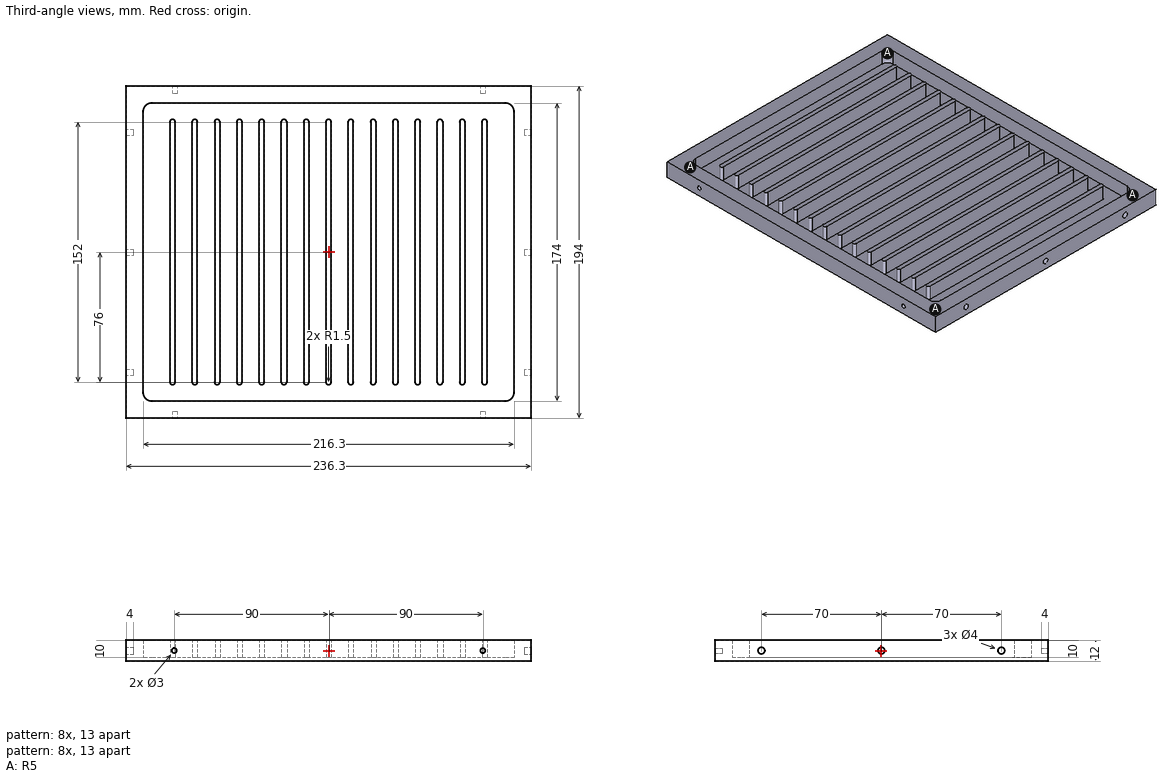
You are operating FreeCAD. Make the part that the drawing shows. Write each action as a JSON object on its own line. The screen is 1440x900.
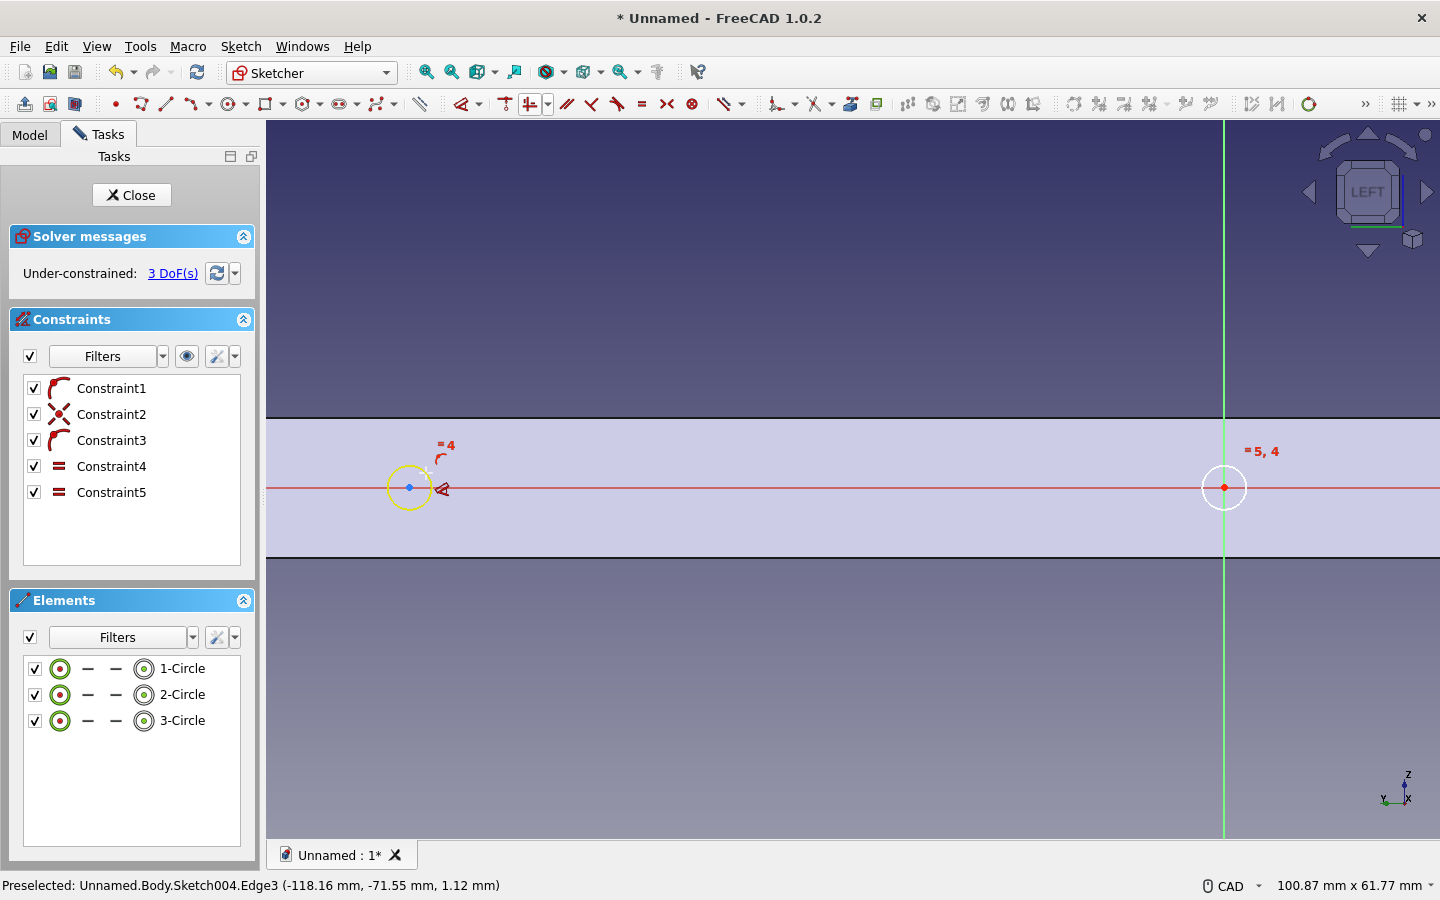
{"action": "left_click", "coordinate": [425, 472]}
{"action": "left_click", "coordinate": [447, 449]}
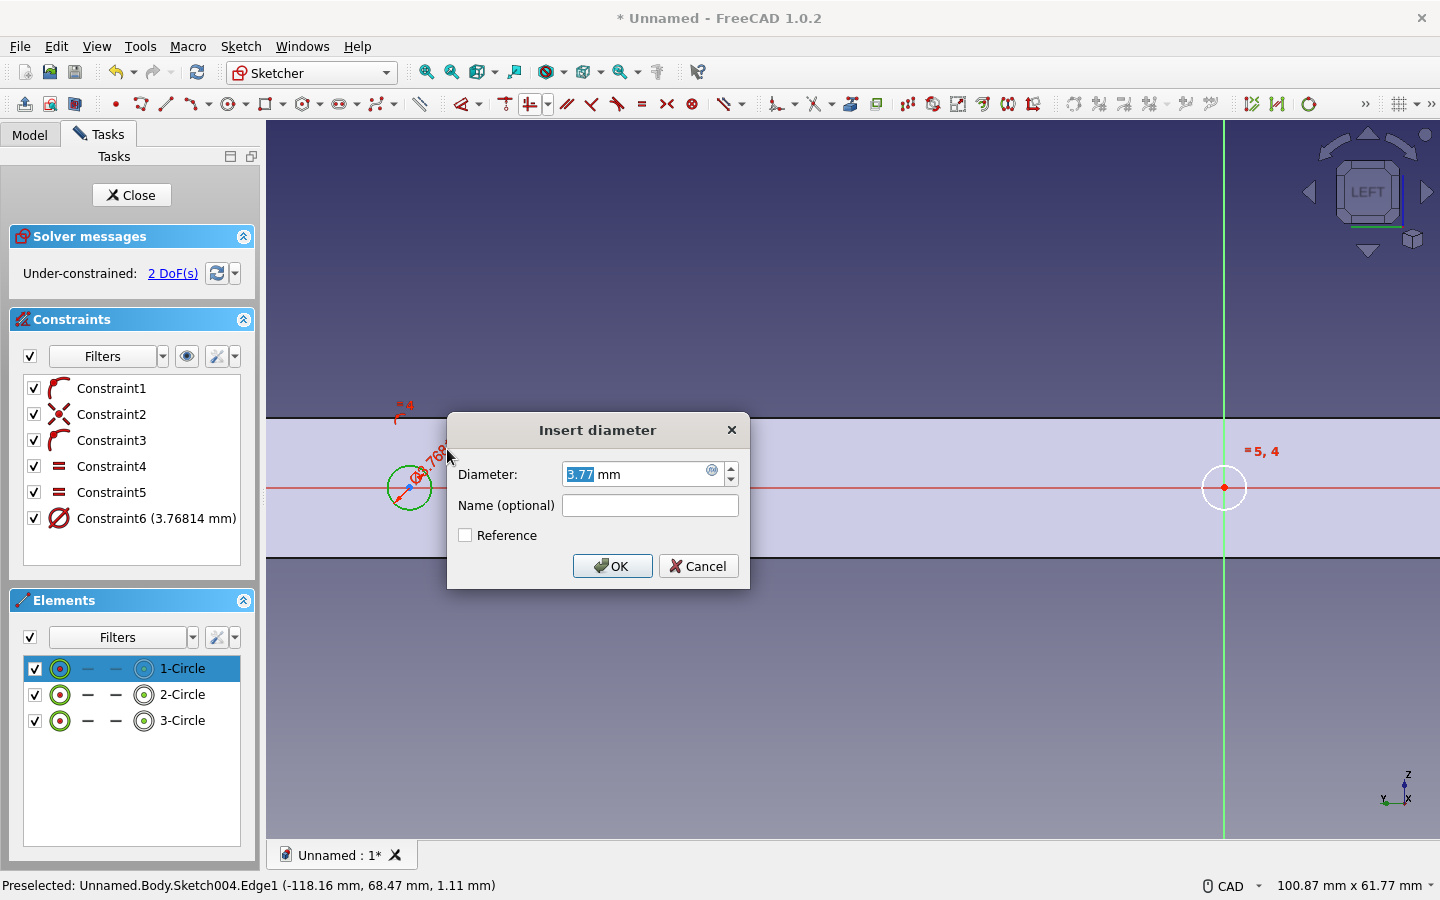
{"action": "type", "text": "4"}
{"action": "key", "text": "Return"}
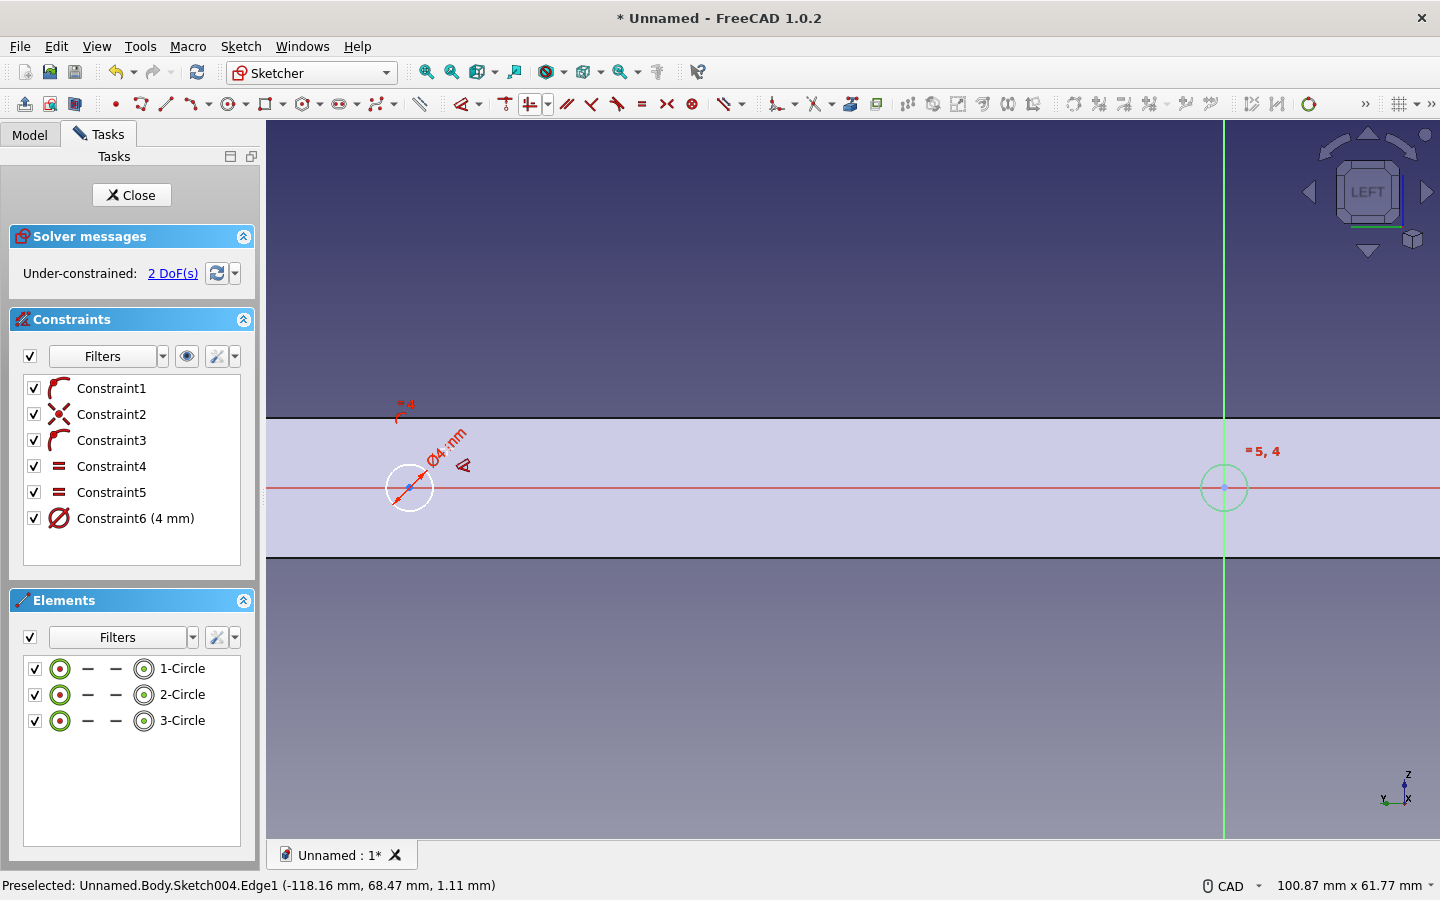
{"action": "left_click", "coordinate": [410, 488]}
{"action": "left_click", "coordinate": [817, 522]}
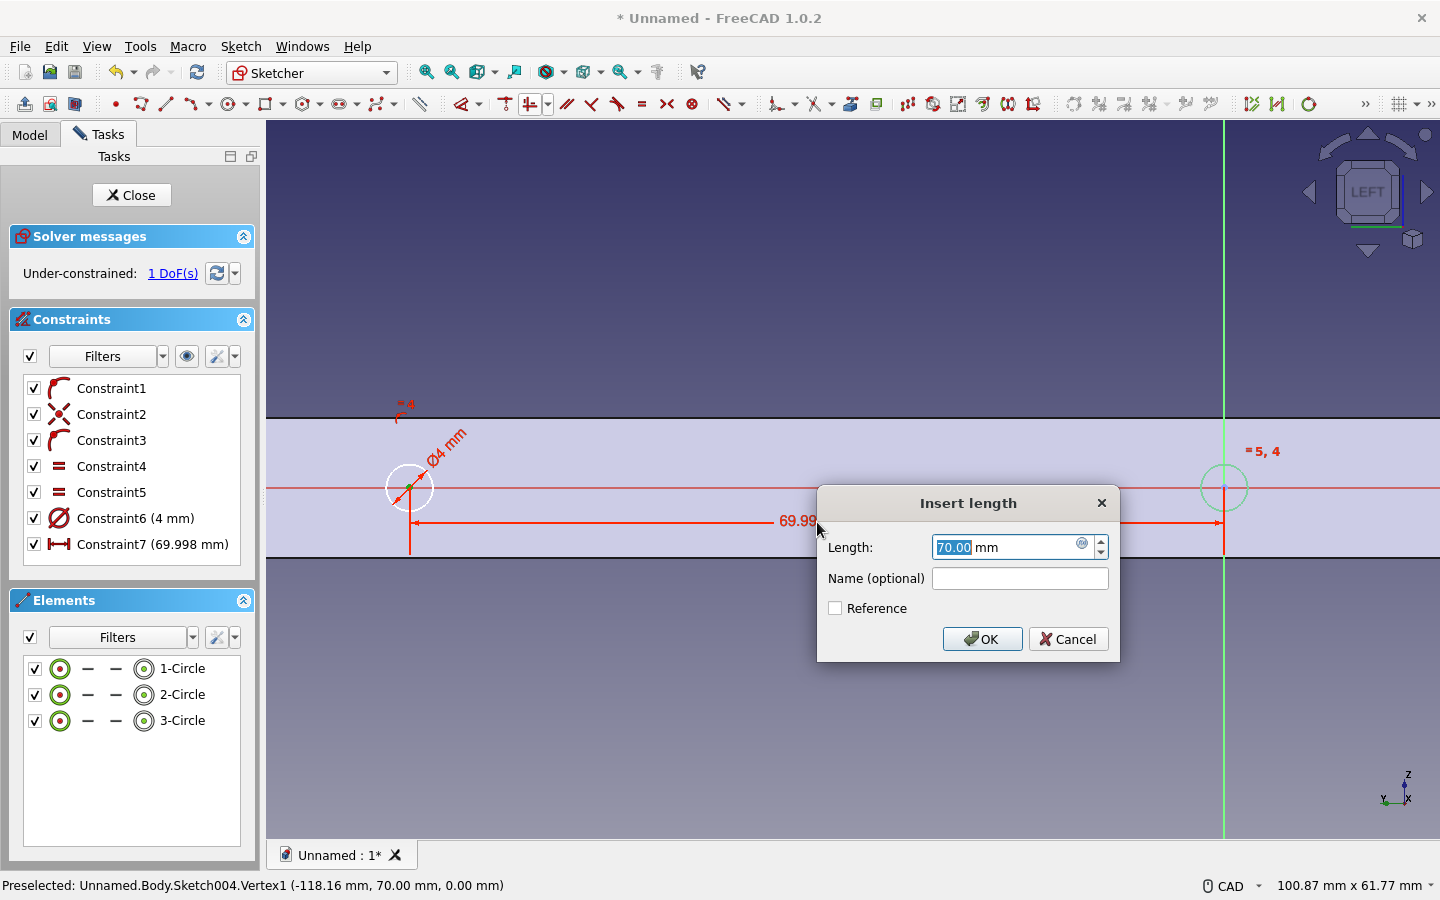
{"action": "type", "text": "70"}
{"action": "key", "text": "Return"}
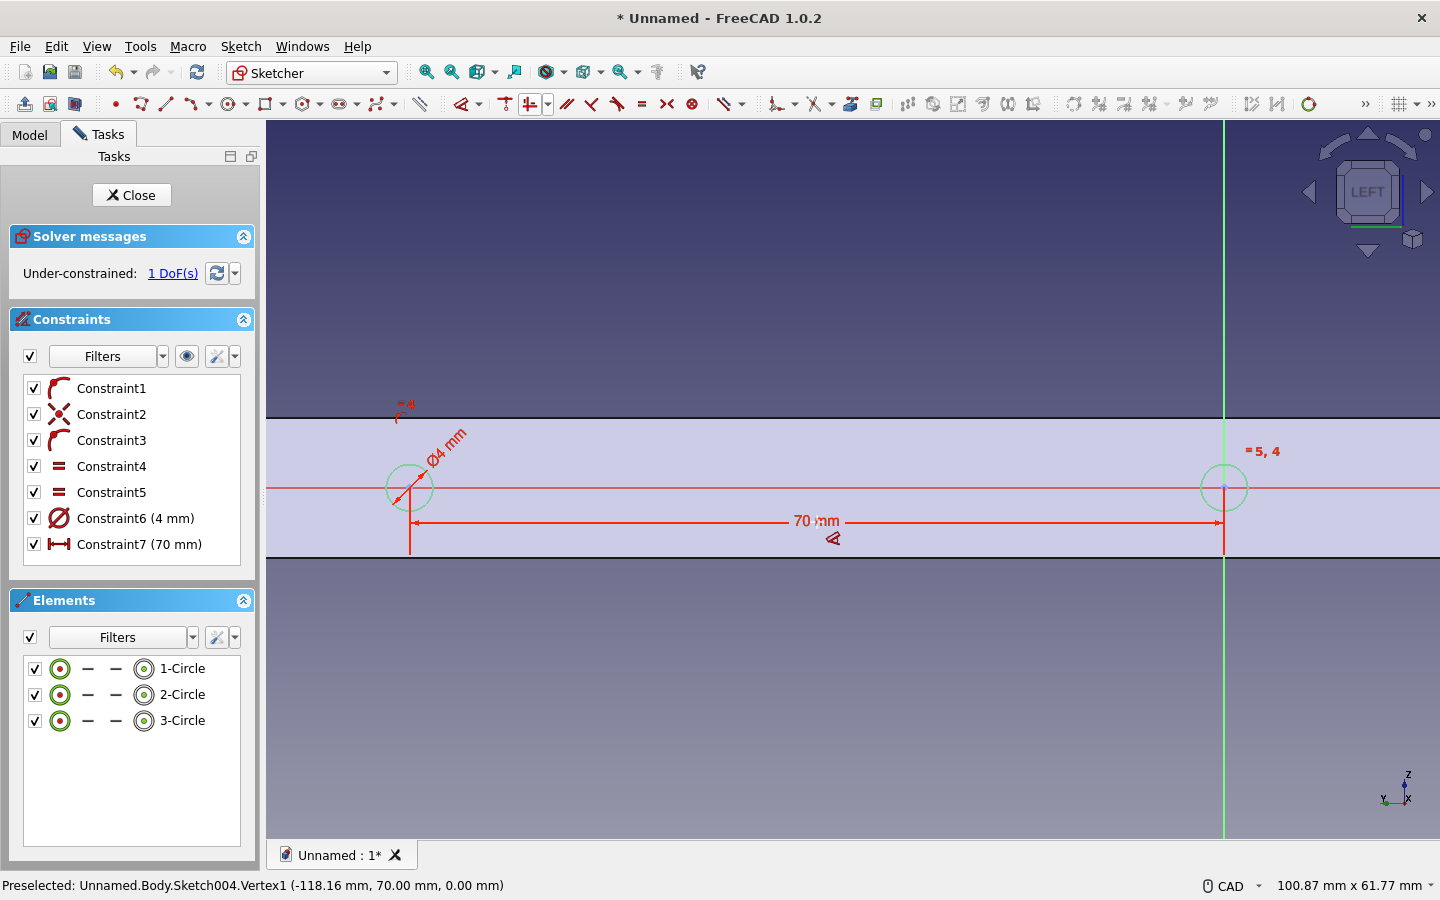
{"action": "scroll", "coordinate": [426, 473], "scroll_direction": "down", "scroll_amount": 4}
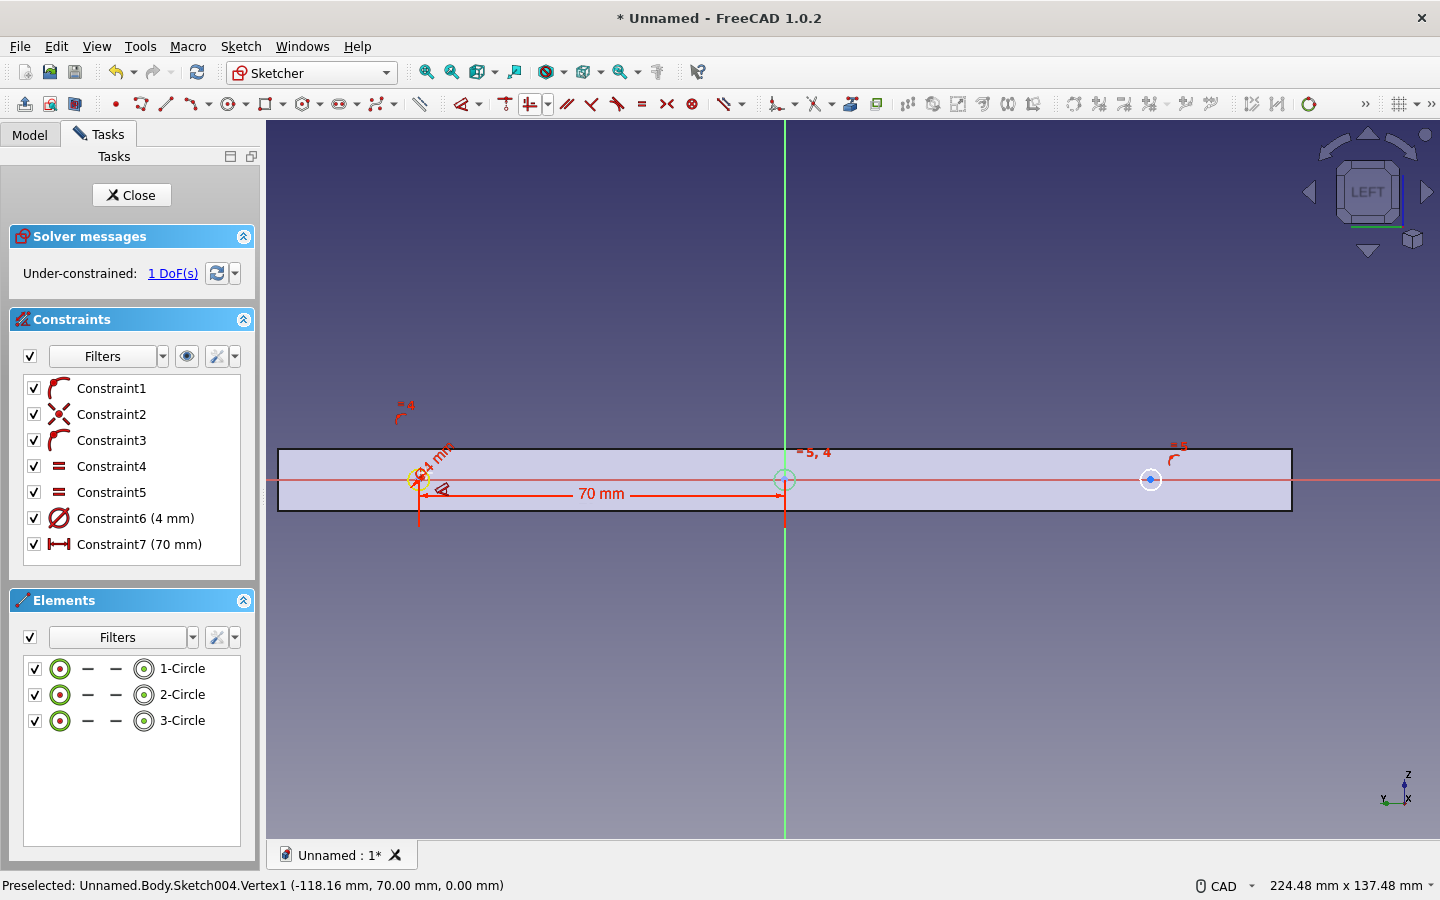
{"action": "left_click", "coordinate": [1151, 480]}
{"action": "left_click", "coordinate": [968, 514]}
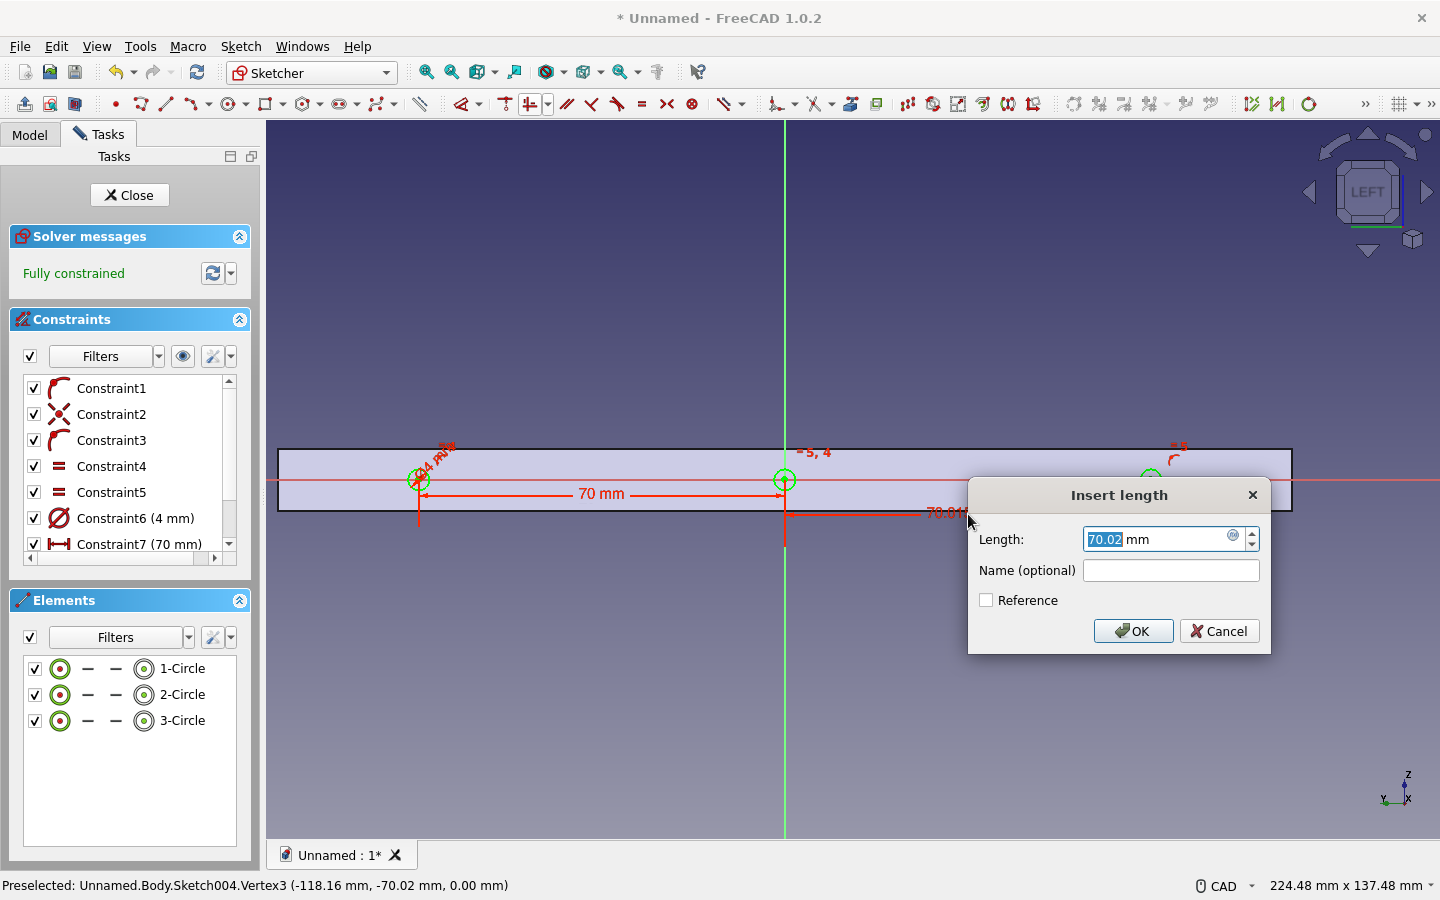
{"action": "type", "text": "70"}
{"action": "key", "text": "Return"}
{"action": "key", "text": "Escape"}